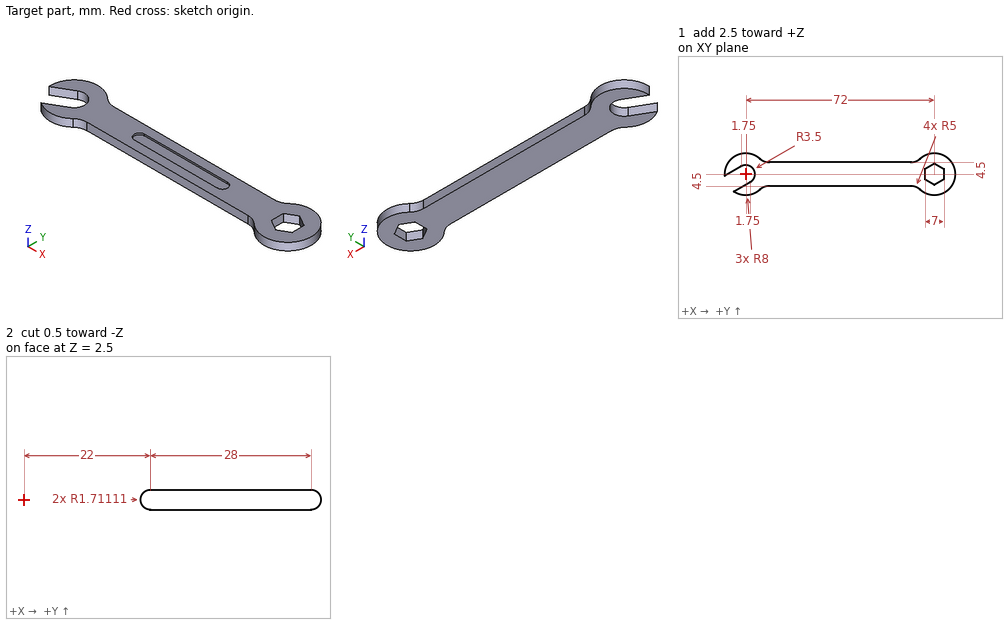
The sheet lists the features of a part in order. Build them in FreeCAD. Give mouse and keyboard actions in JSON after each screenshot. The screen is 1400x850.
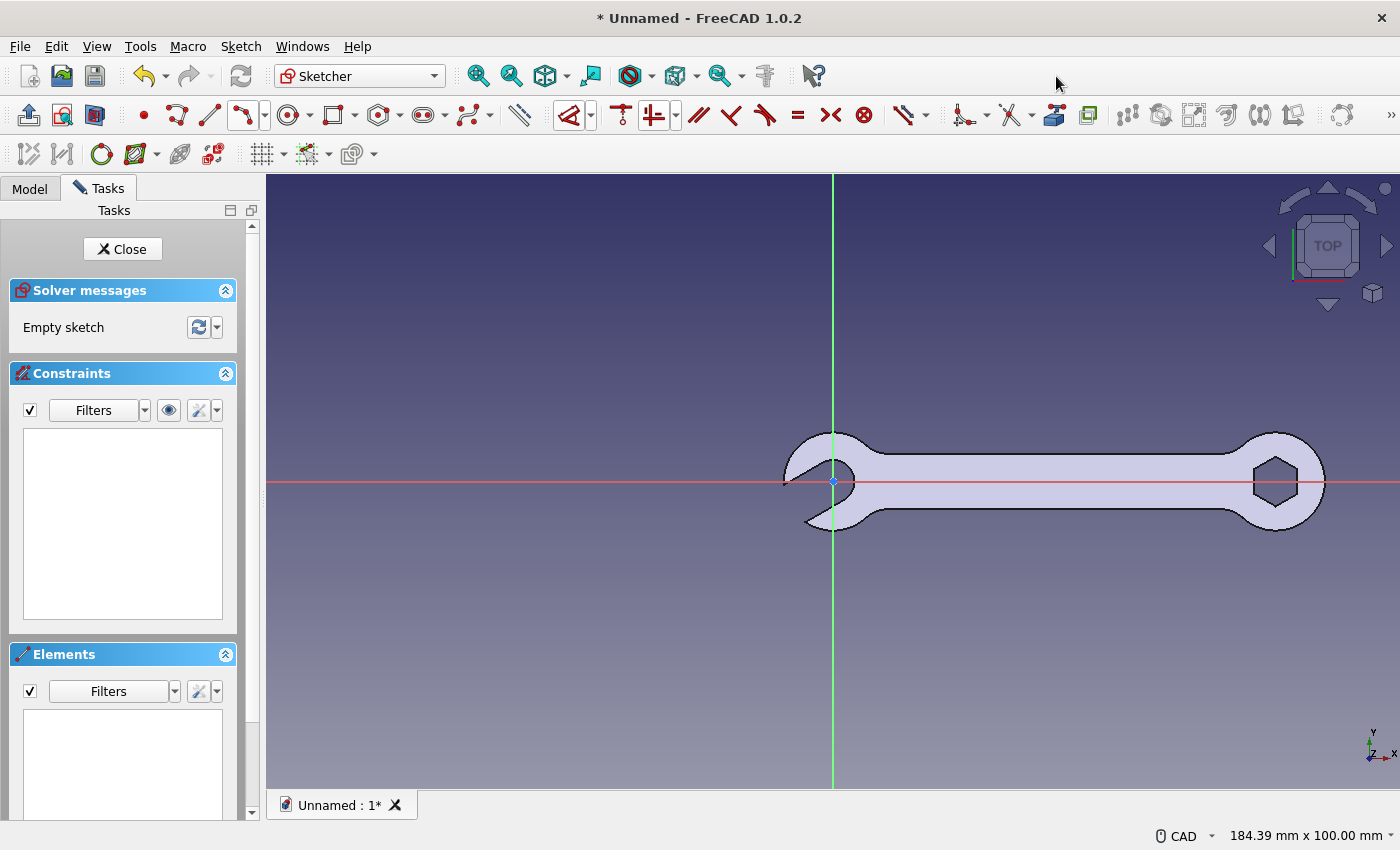
{"action": "scroll", "coordinate": [1178, 482], "scroll_direction": "up", "scroll_amount": 4}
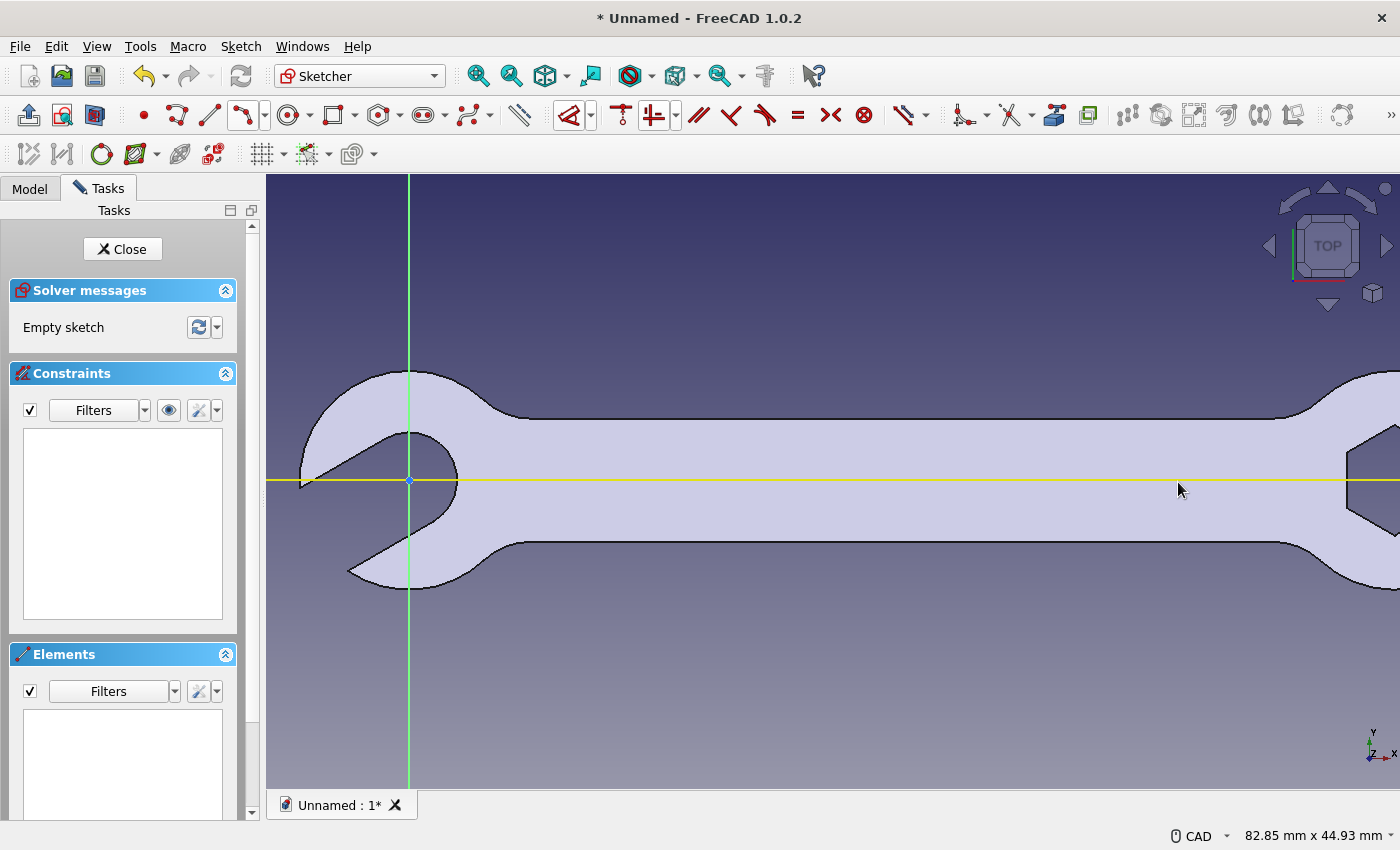
{"action": "left_click", "coordinate": [422, 116]}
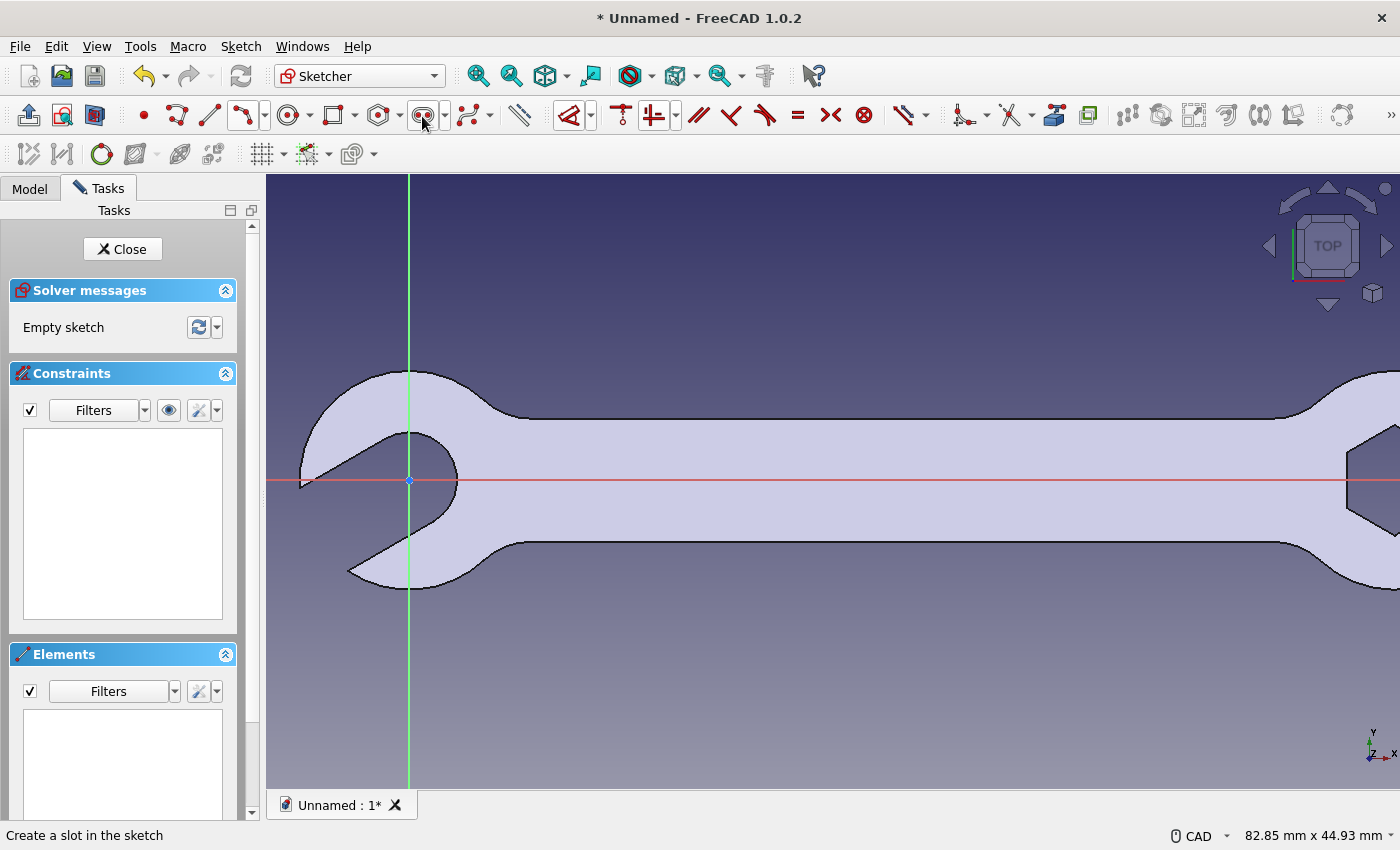
{"action": "left_click", "coordinate": [710, 480]}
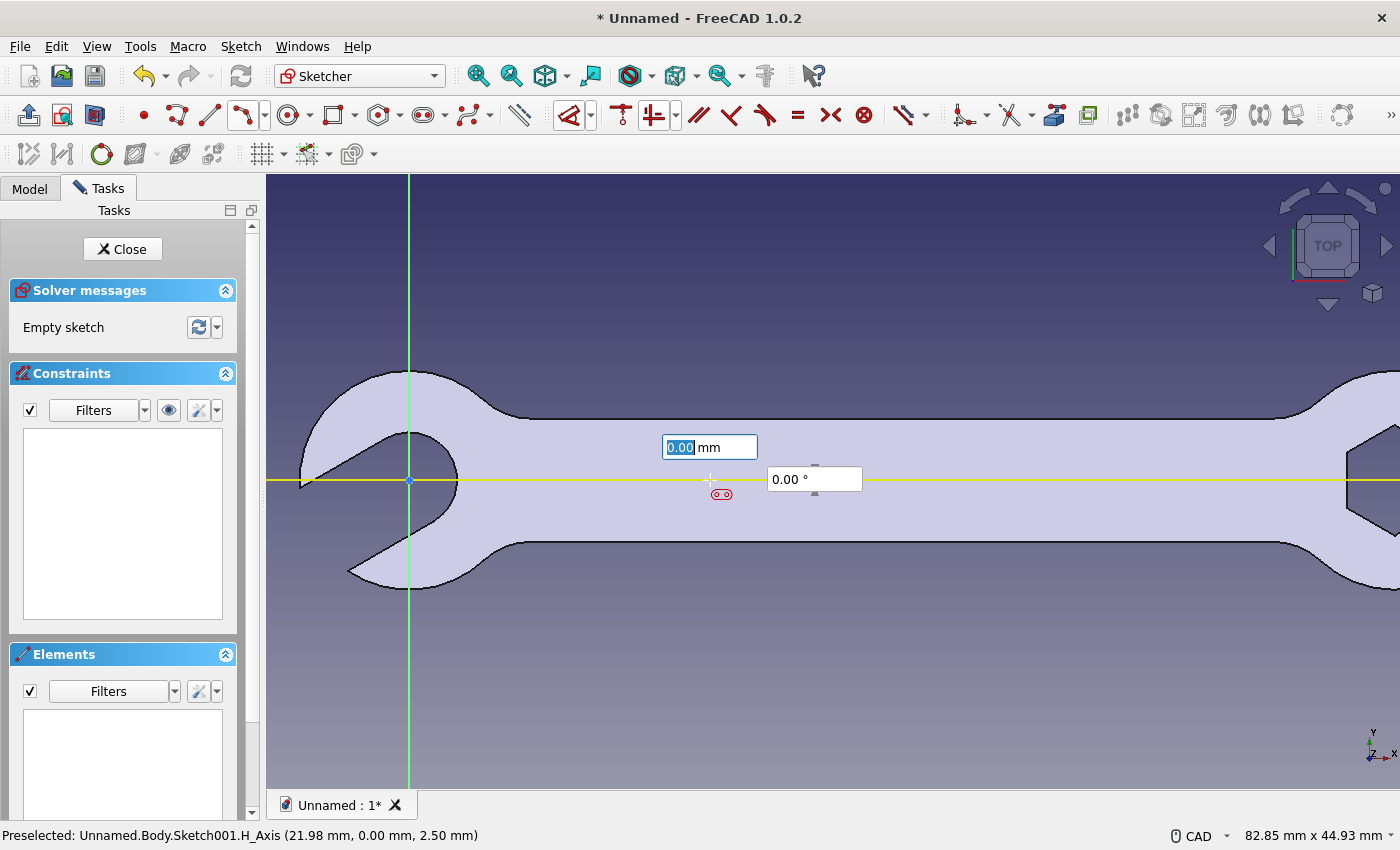
{"action": "left_click", "coordinate": [1094, 471]}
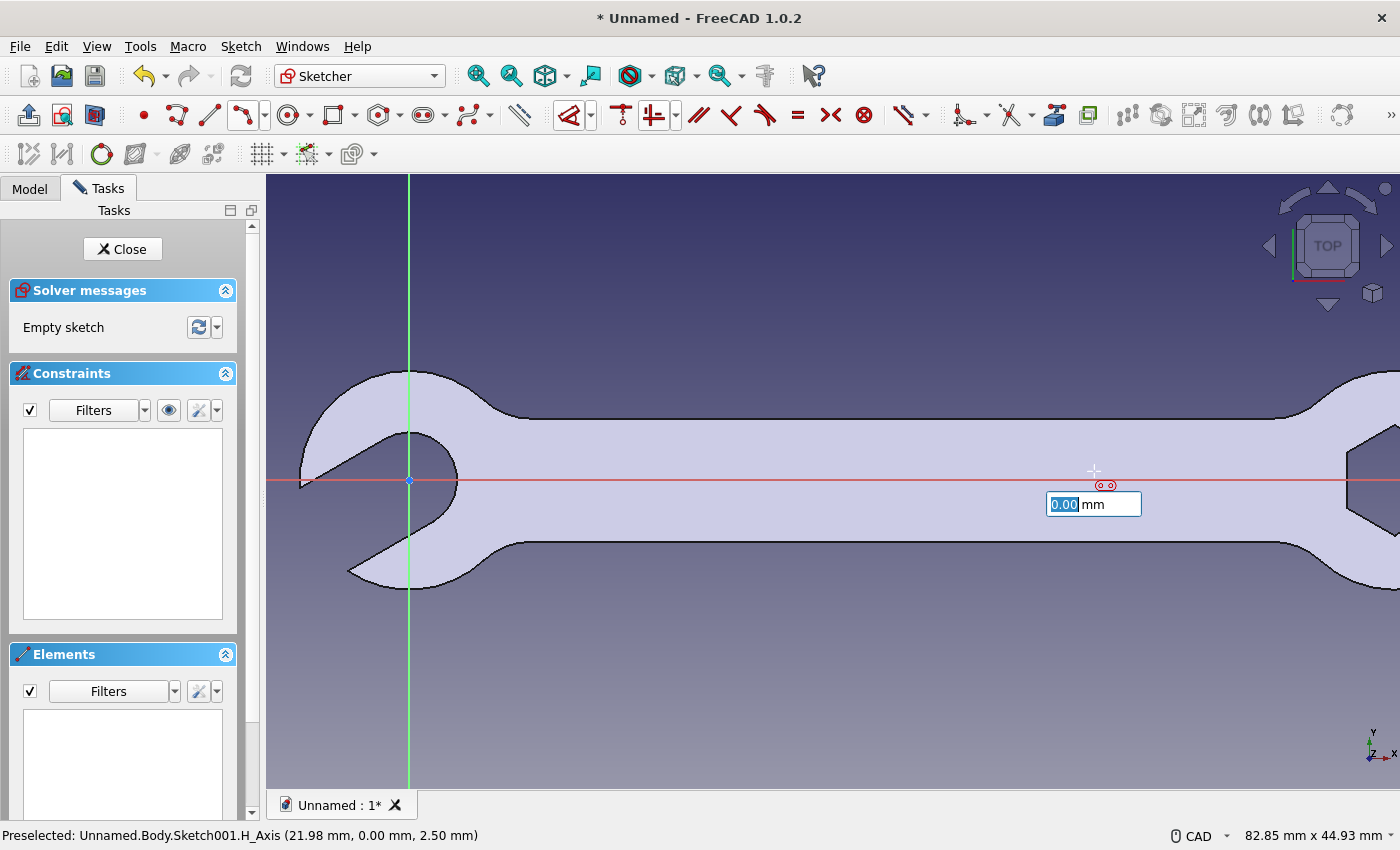
{"action": "left_click", "coordinate": [902, 457]}
{"action": "key", "text": "Escape"}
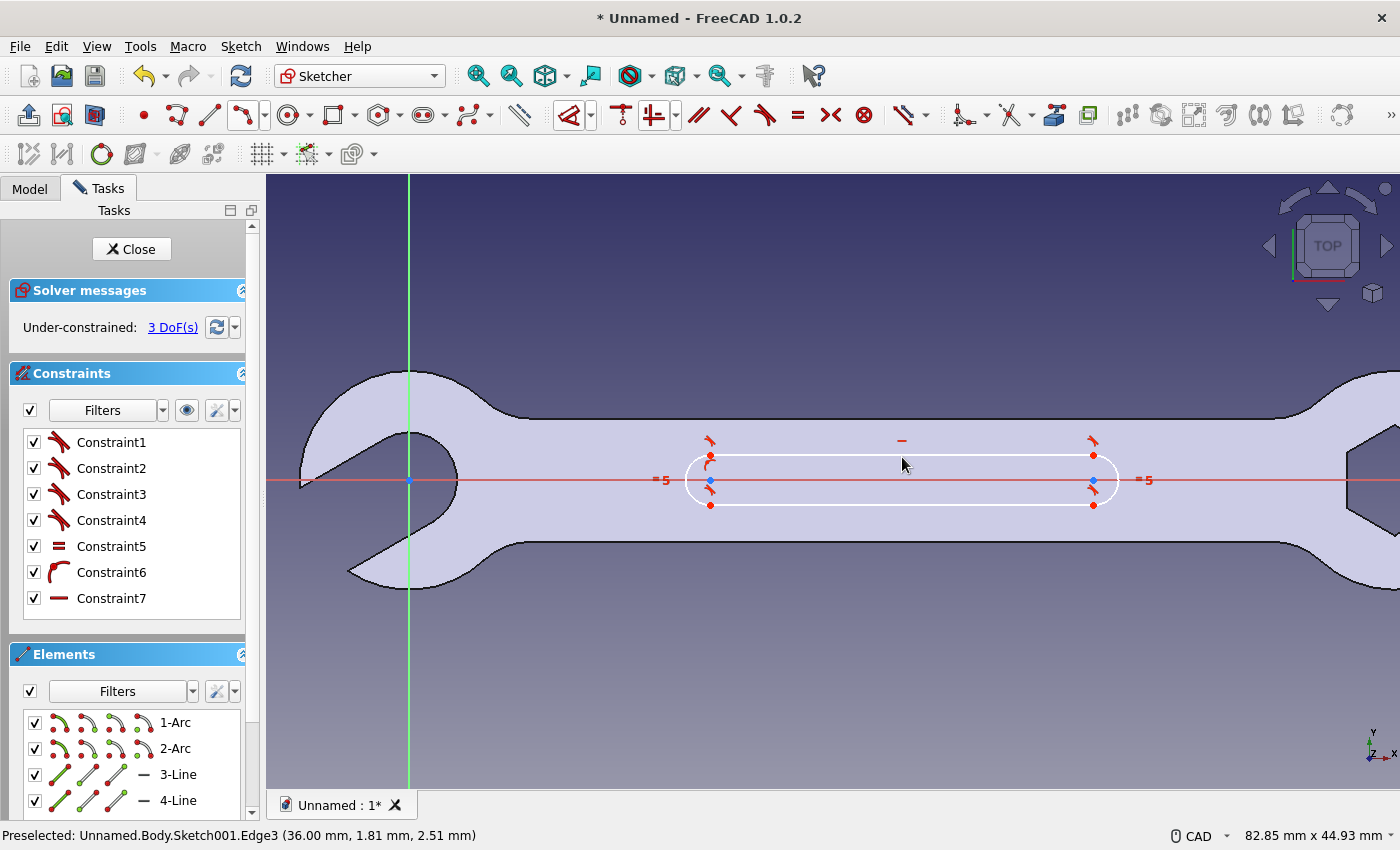
{"action": "scroll", "coordinate": [690, 466], "scroll_direction": "up", "scroll_amount": 3}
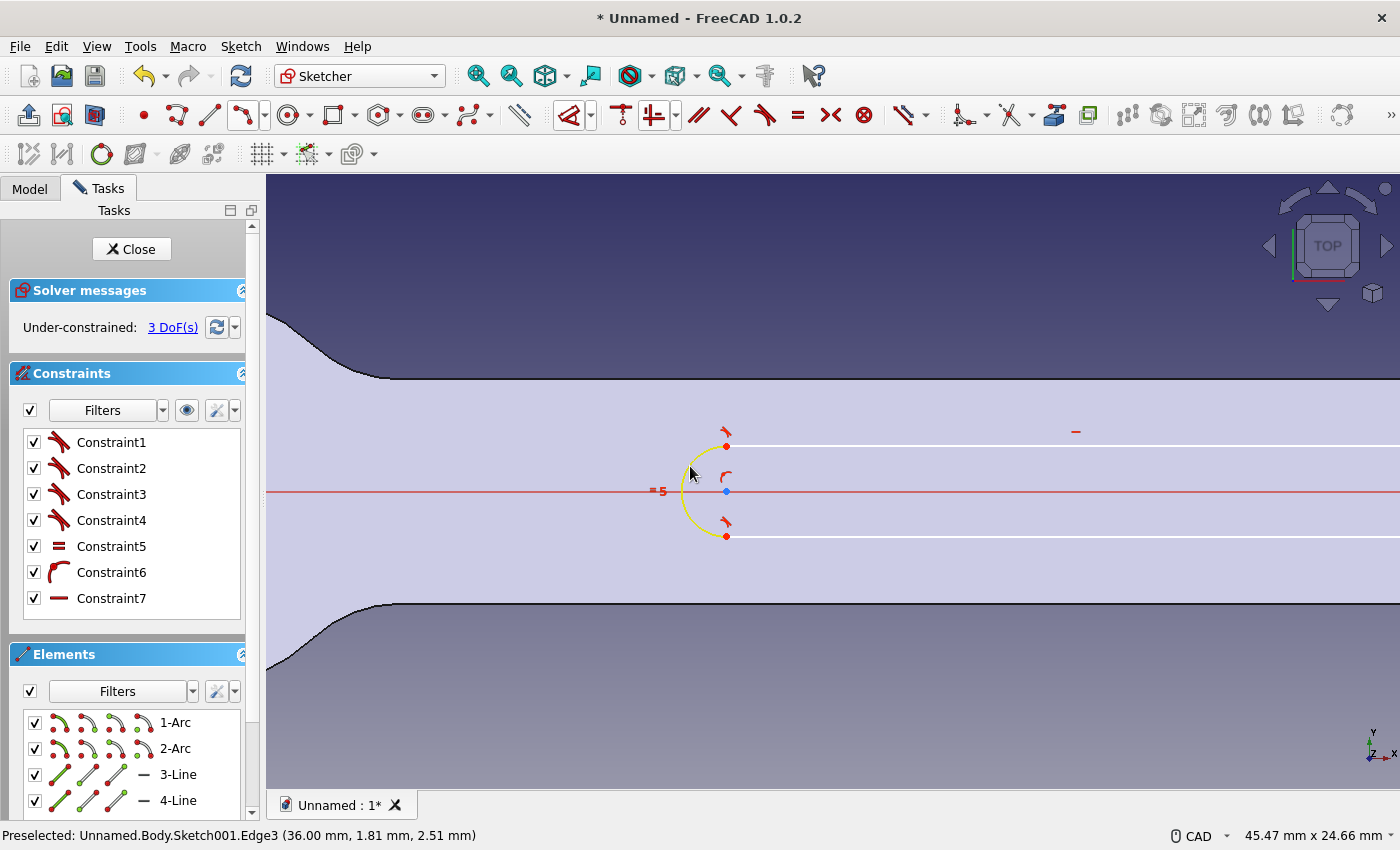
{"action": "left_click", "coordinate": [690, 465]}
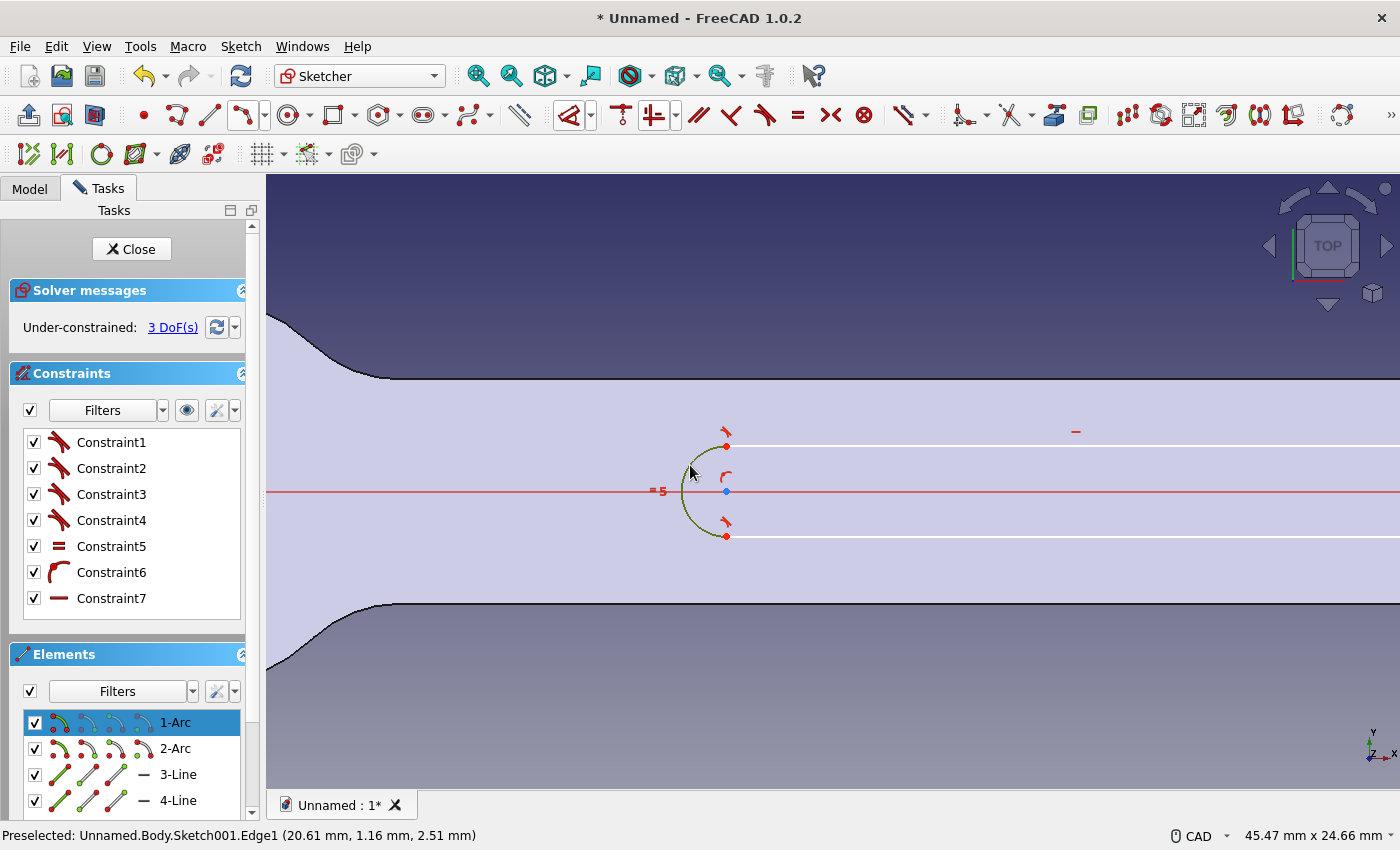
{"action": "left_click", "coordinate": [590, 116]}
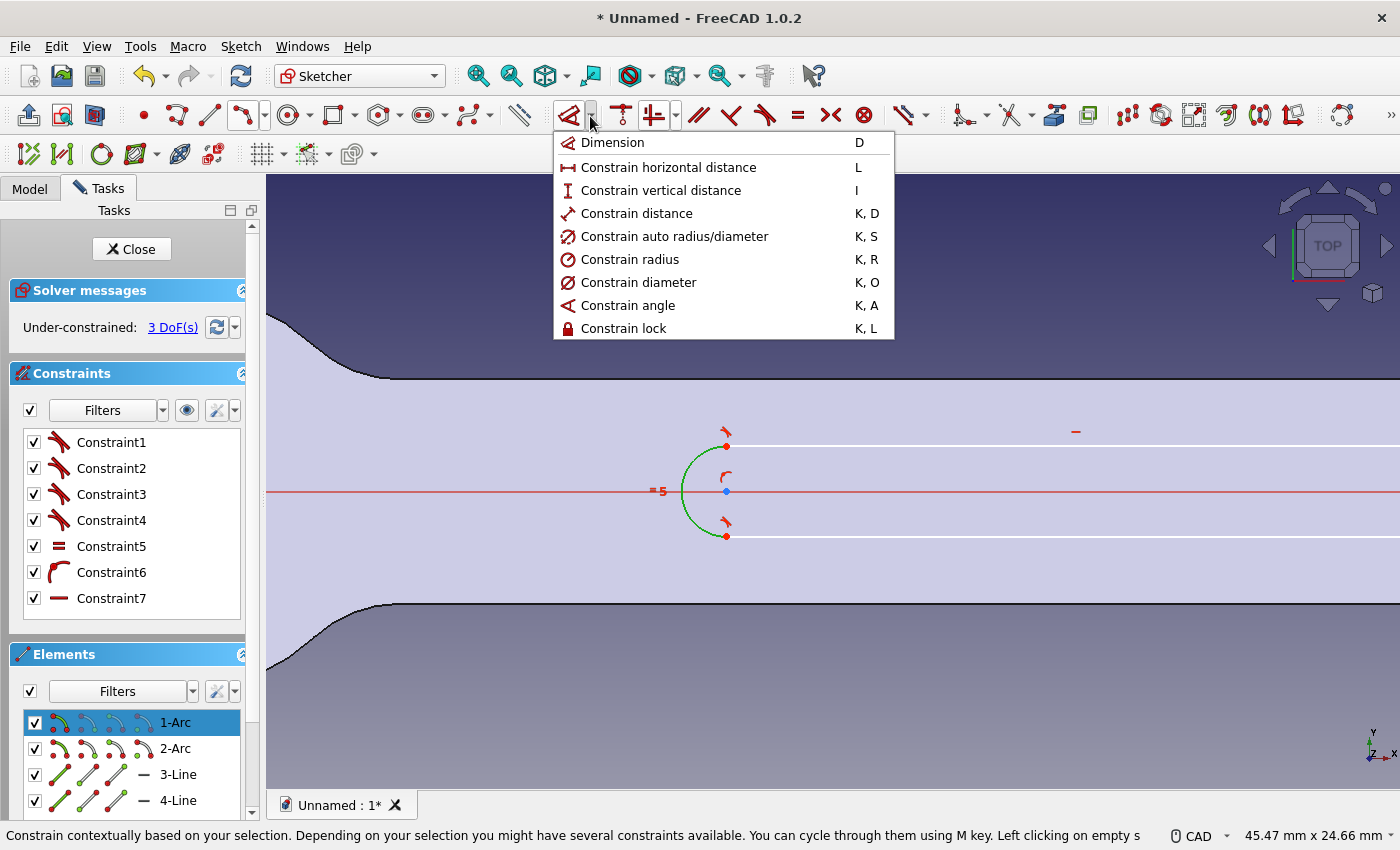
{"action": "left_click", "coordinate": [724, 260]}